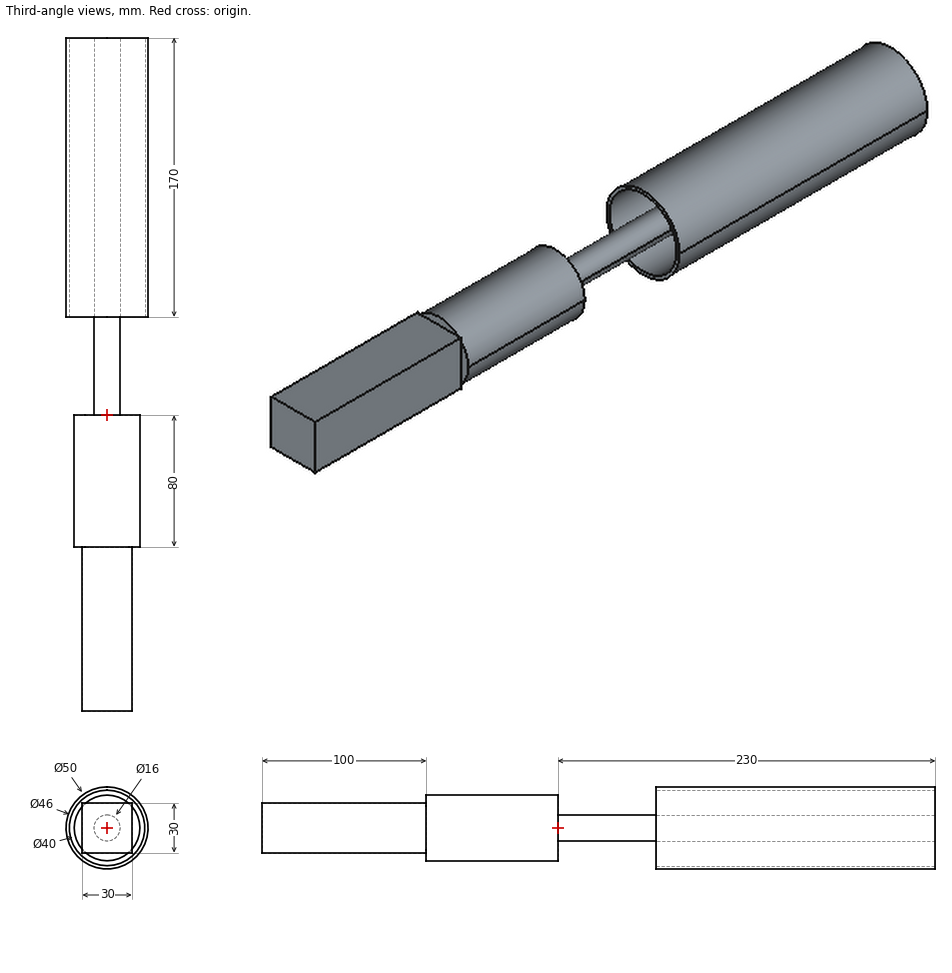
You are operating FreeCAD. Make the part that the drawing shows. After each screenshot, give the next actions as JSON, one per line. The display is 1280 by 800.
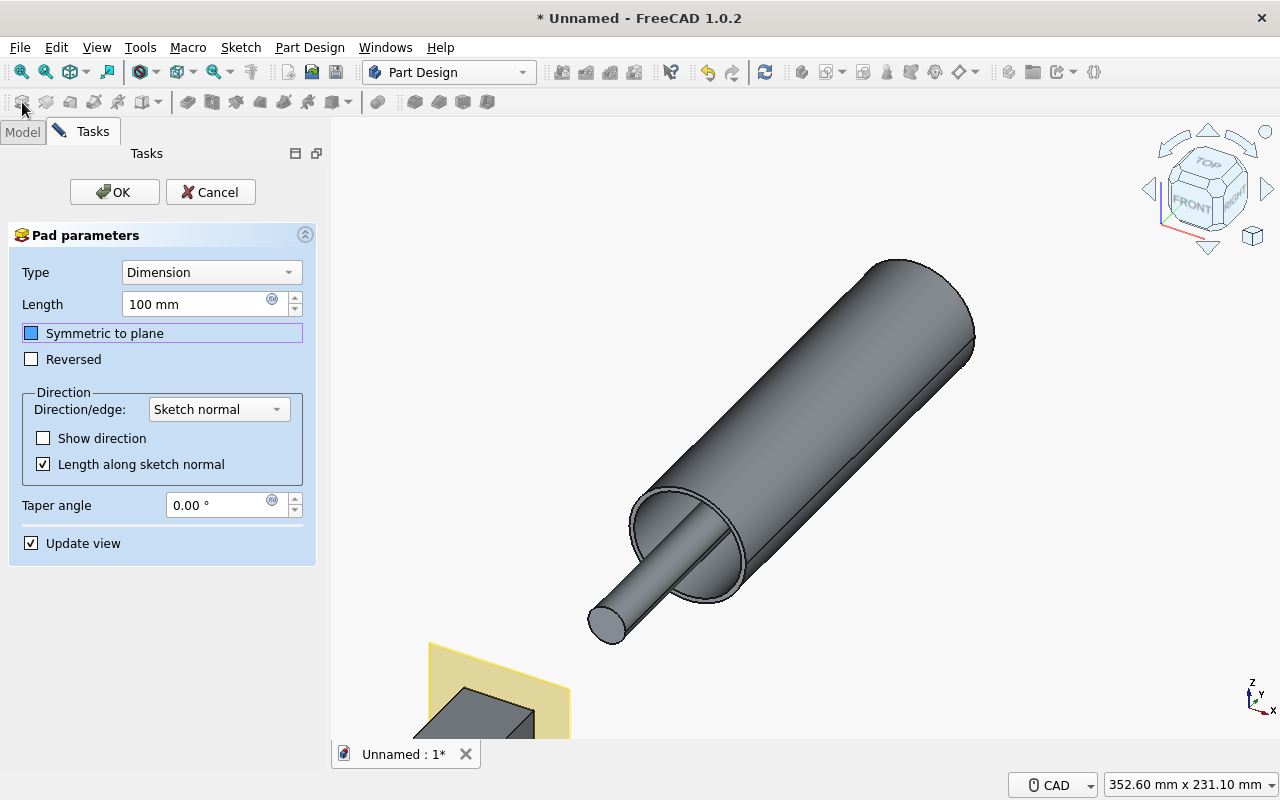
{"action": "left_click", "coordinate": [115, 192]}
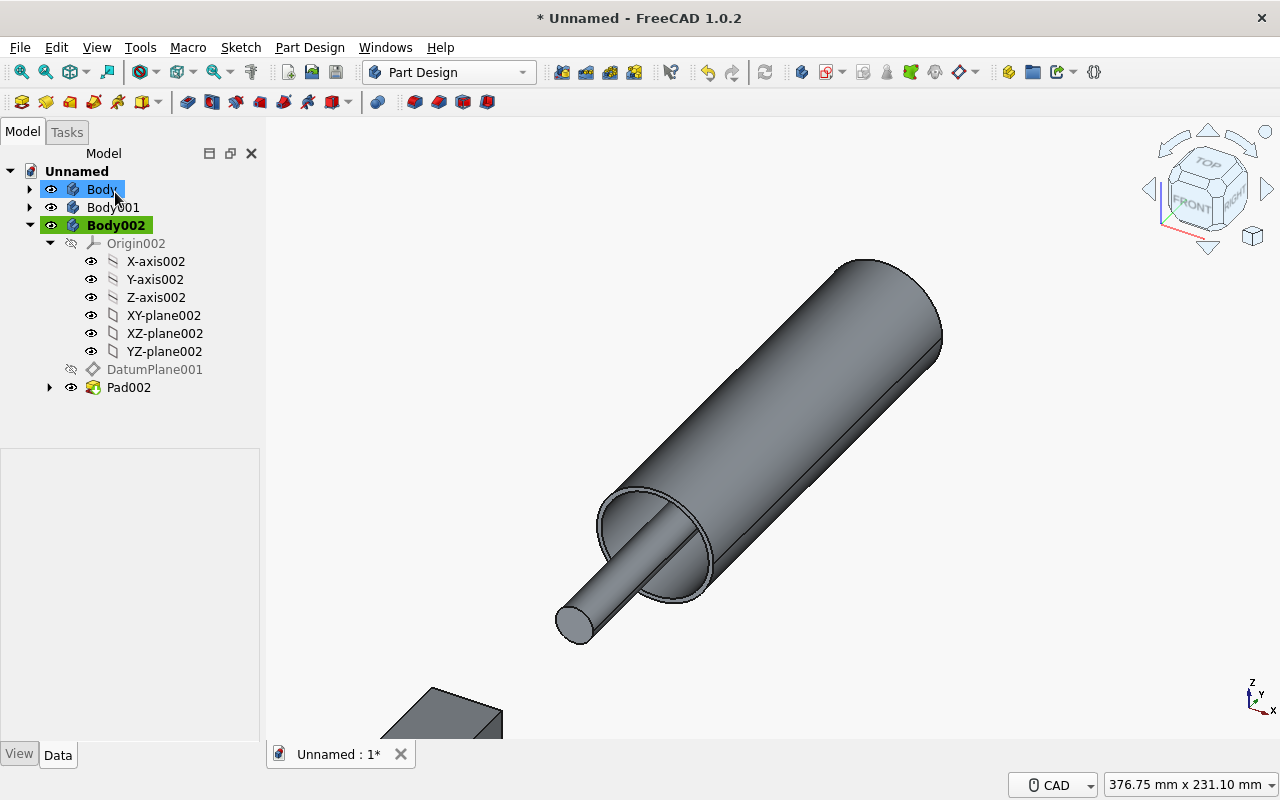
{"action": "left_click", "coordinate": [22, 72]}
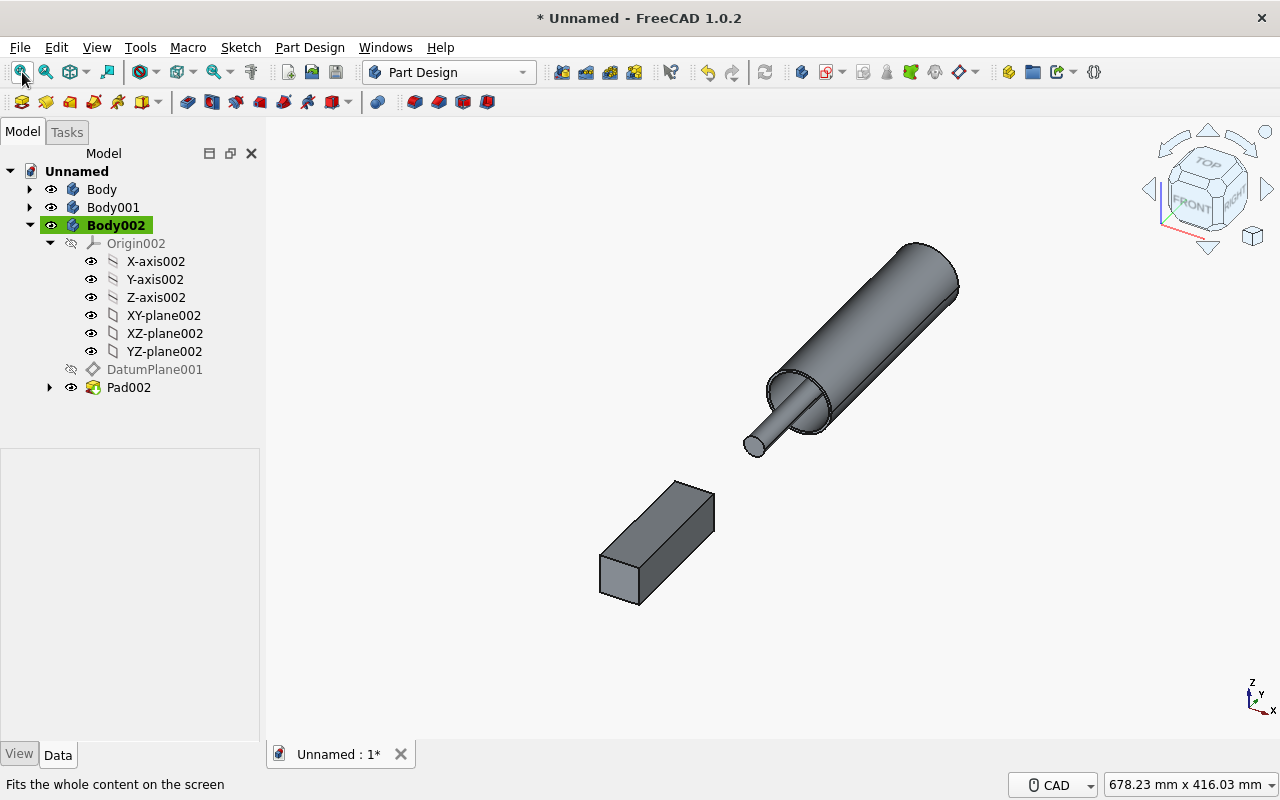
{"action": "double_click", "coordinate": [96, 189]}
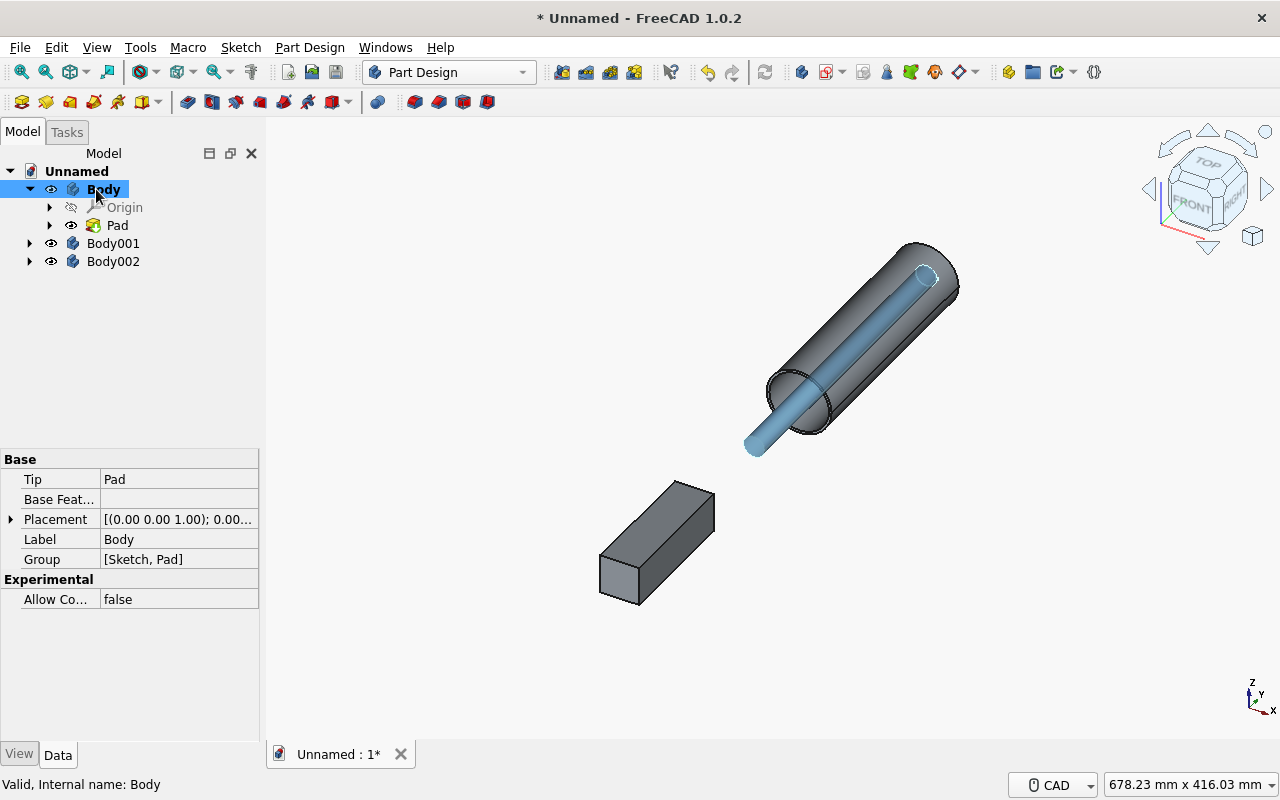
{"action": "left_click", "coordinate": [96, 189]}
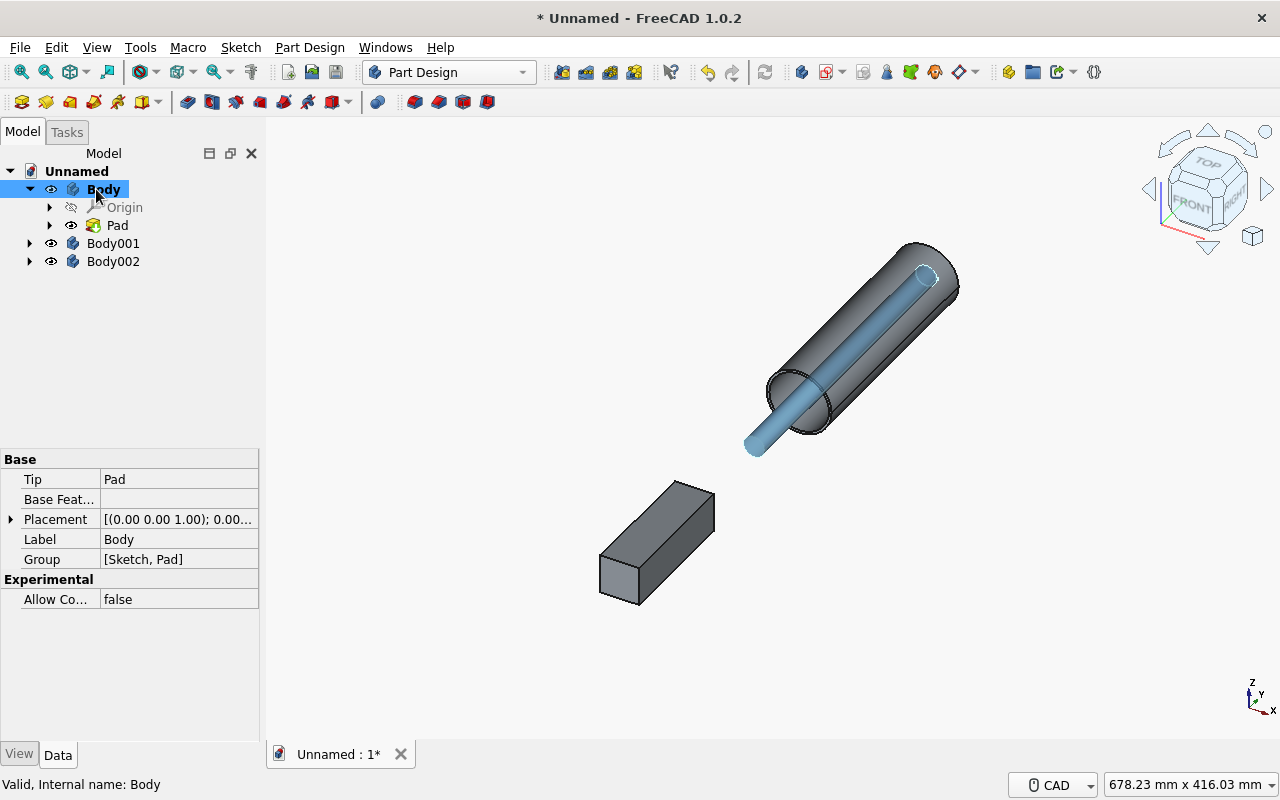
{"action": "left_click", "coordinate": [146, 599]}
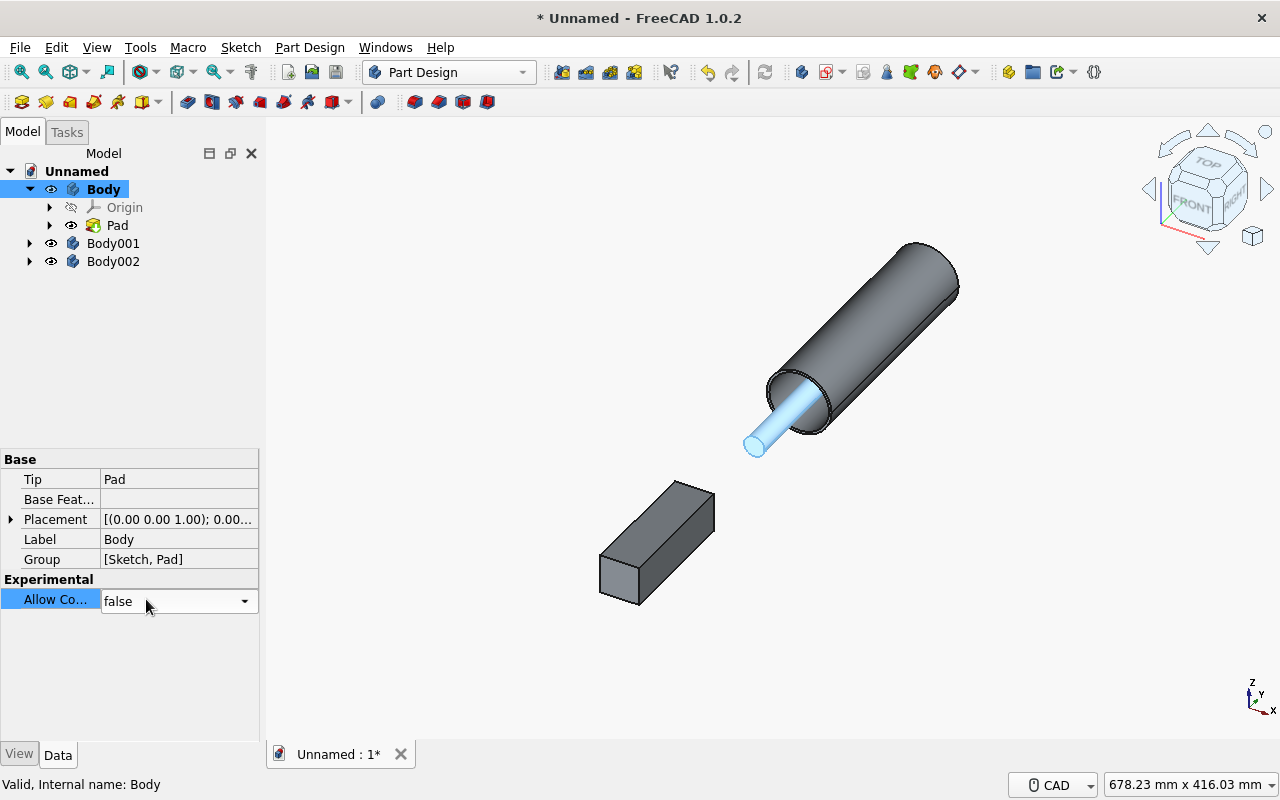
{"action": "left_click", "coordinate": [146, 599]}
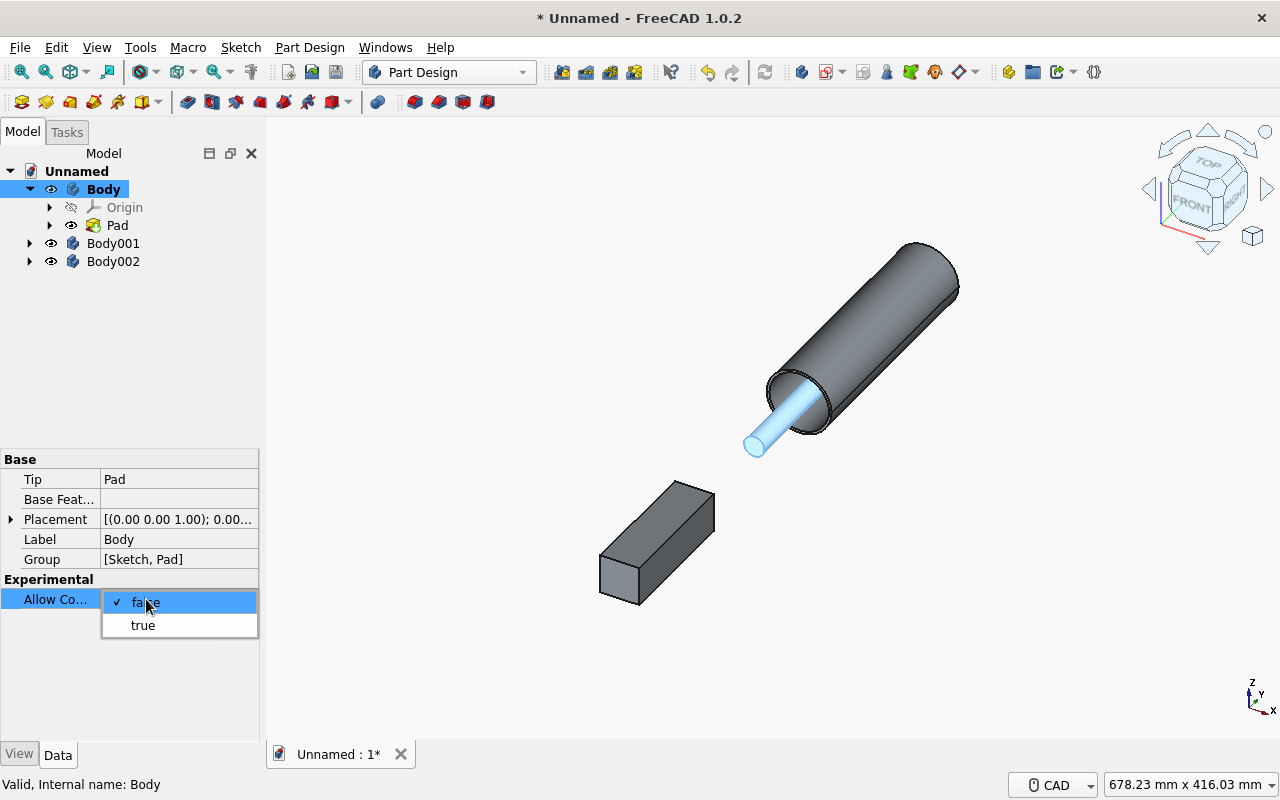
{"action": "left_click", "coordinate": [179, 626]}
{"action": "key", "text": "Return"}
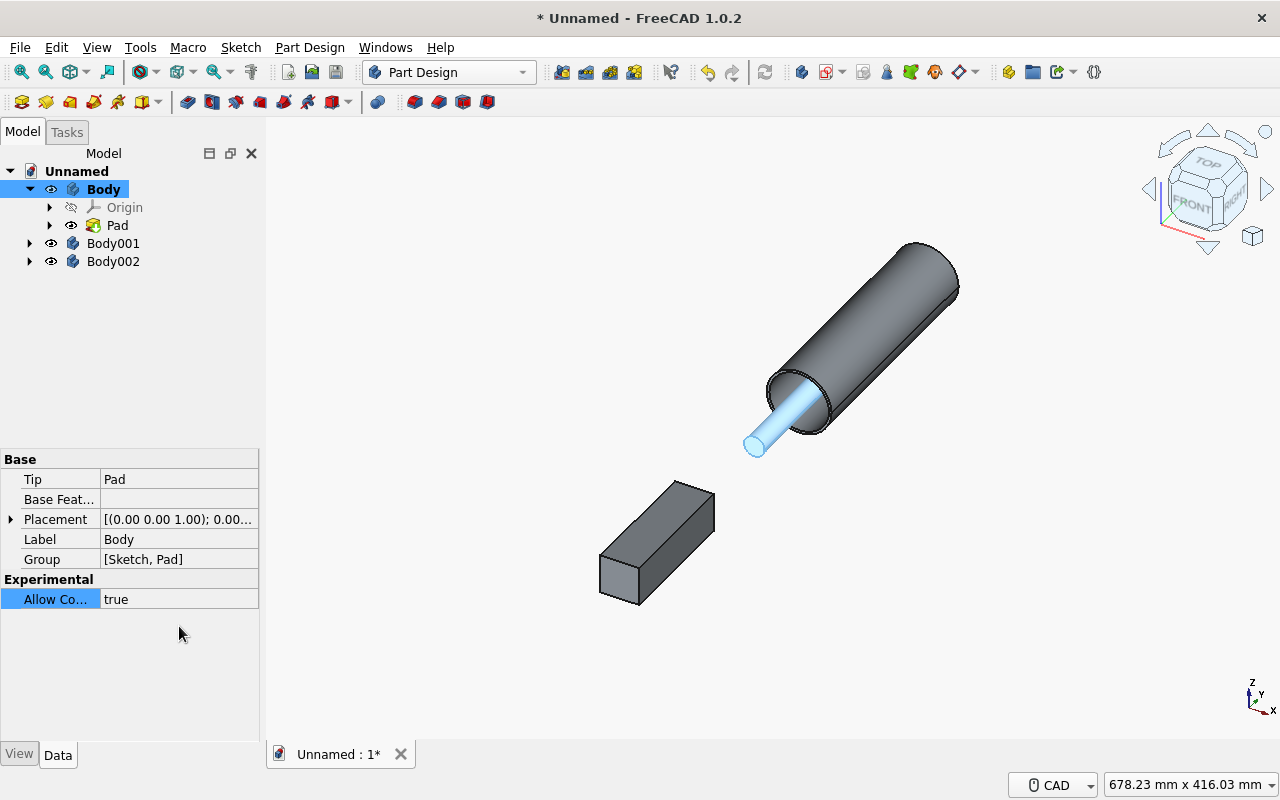
{"action": "left_click", "coordinate": [96, 261]}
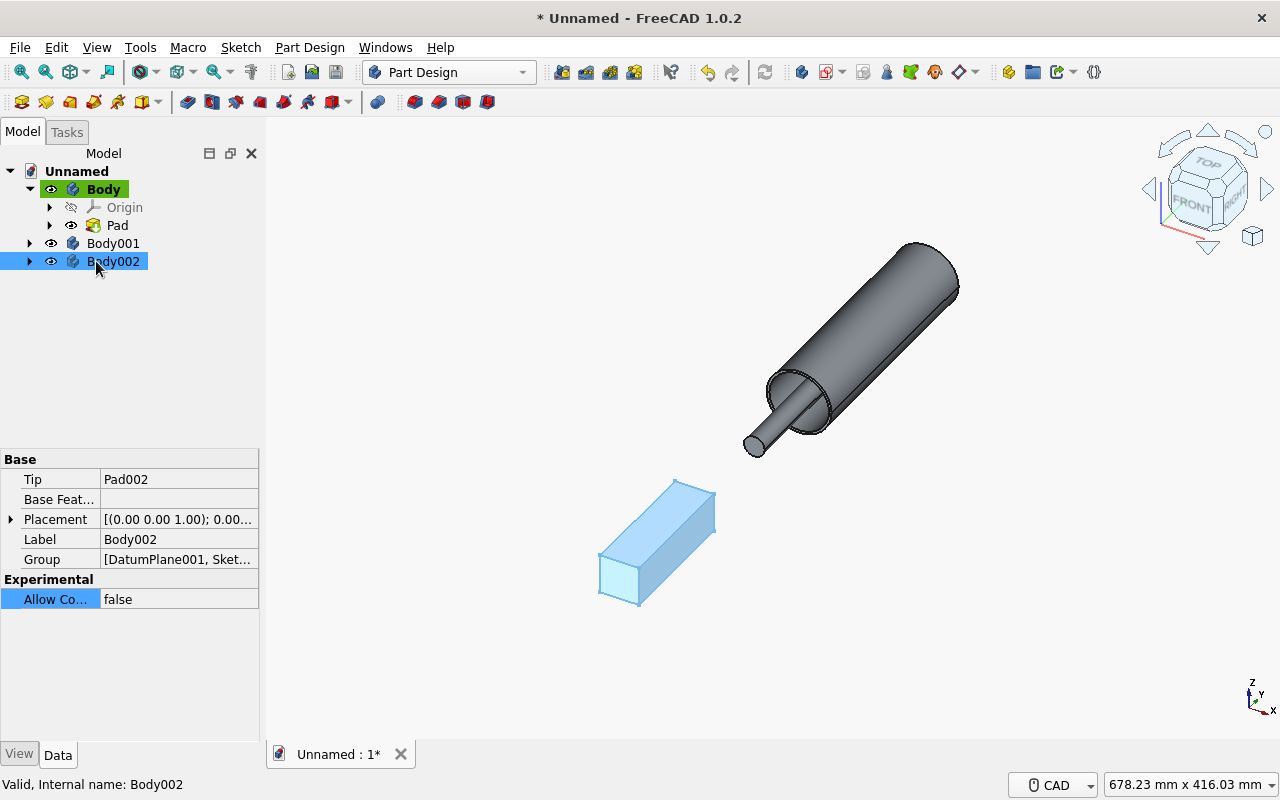
{"action": "left_click", "coordinate": [378, 102]}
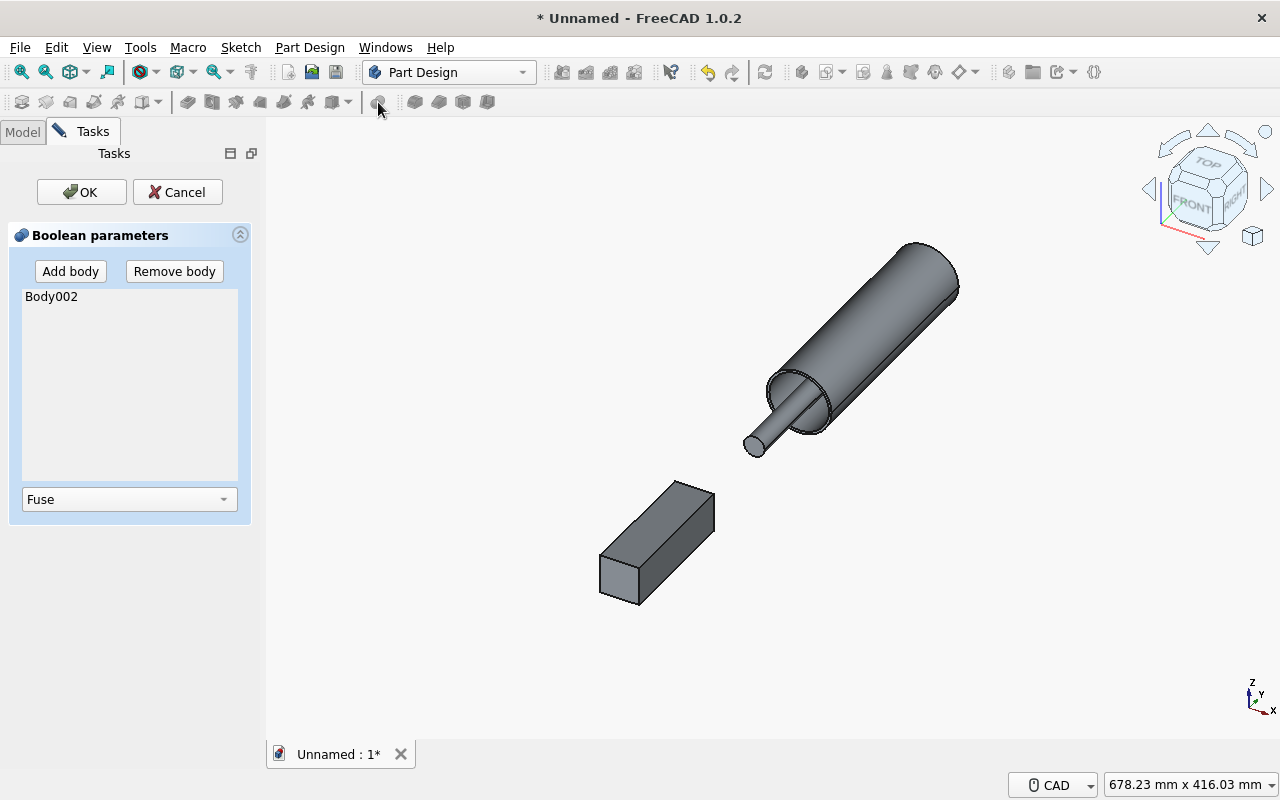
{"action": "left_click", "coordinate": [82, 192]}